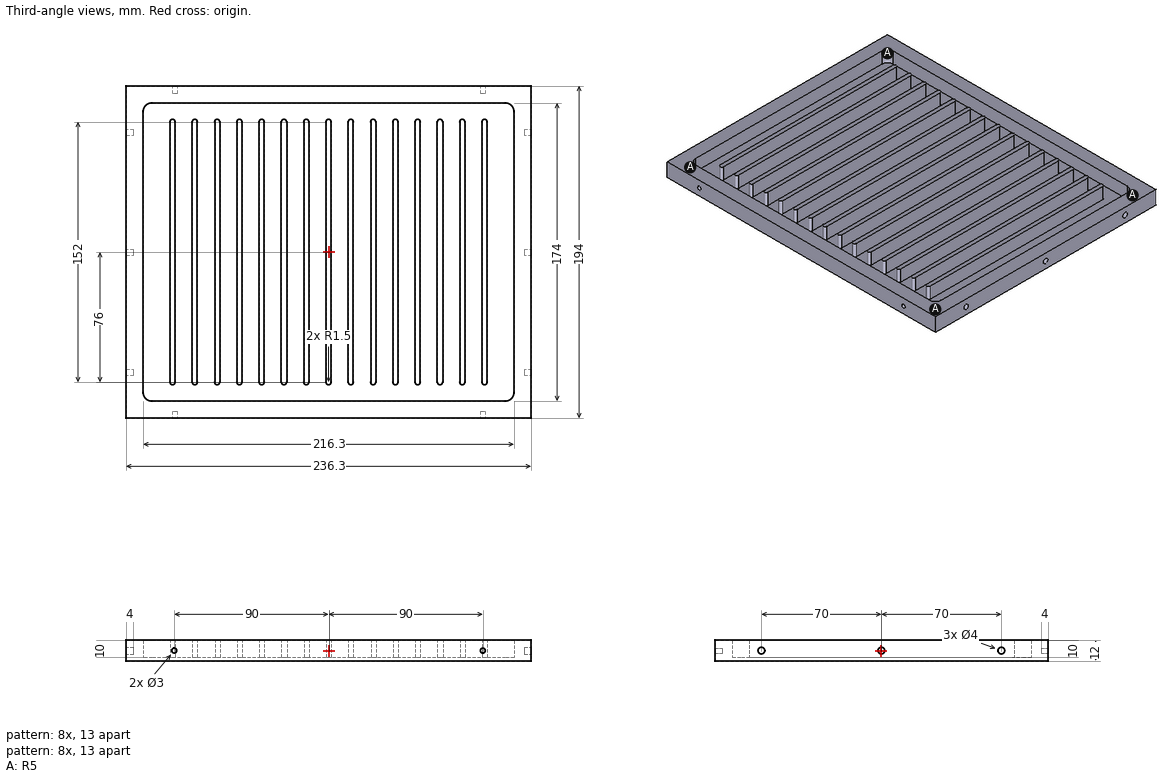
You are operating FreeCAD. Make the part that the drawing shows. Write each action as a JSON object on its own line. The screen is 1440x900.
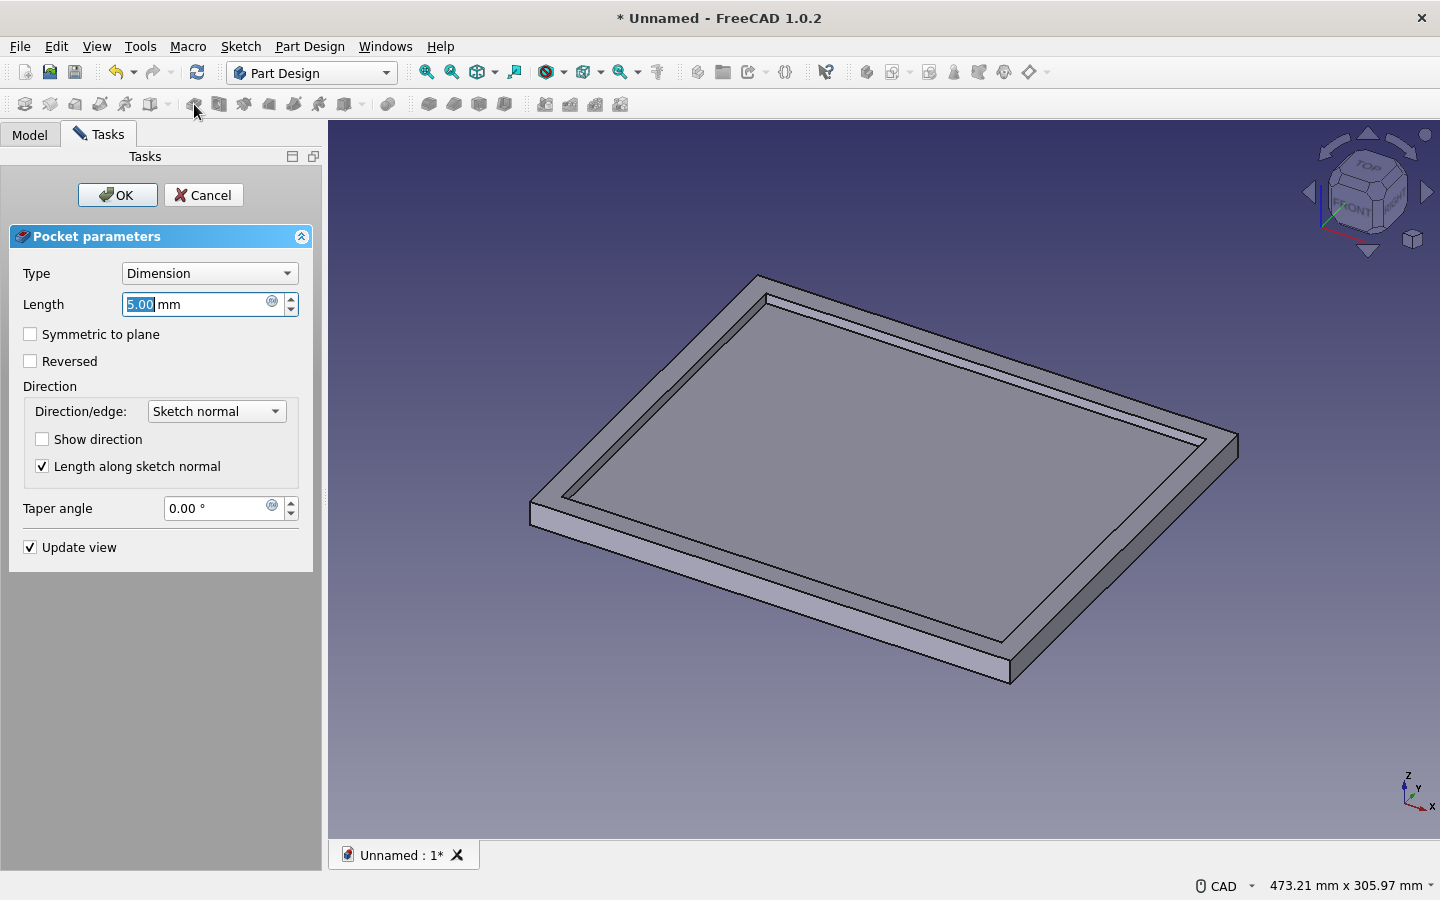
{"action": "type", "text": "10"}
{"action": "key", "text": "Tab"}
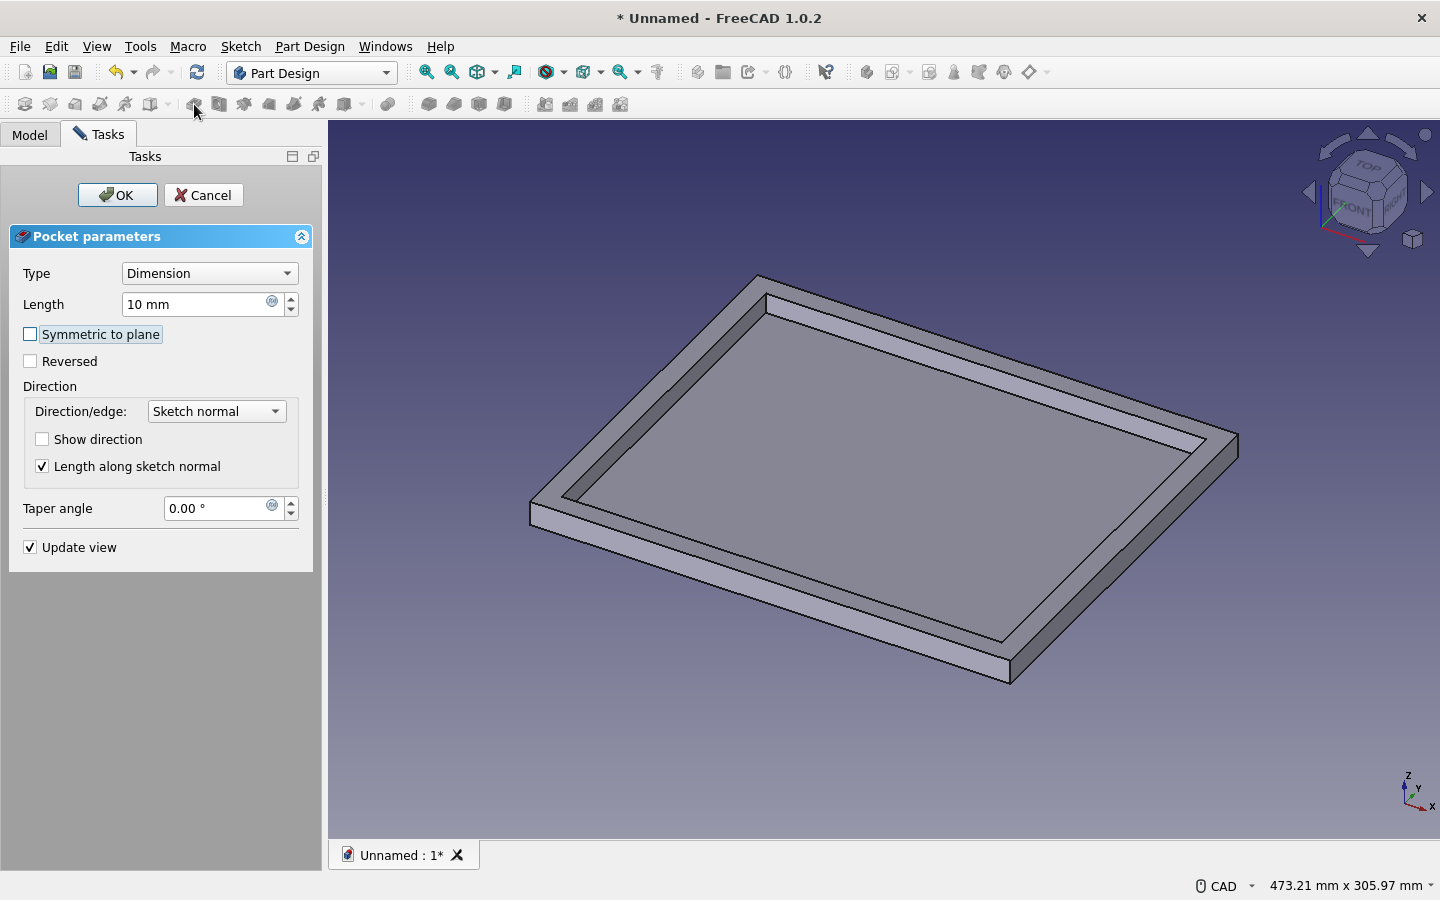
{"action": "left_click", "coordinate": [118, 195]}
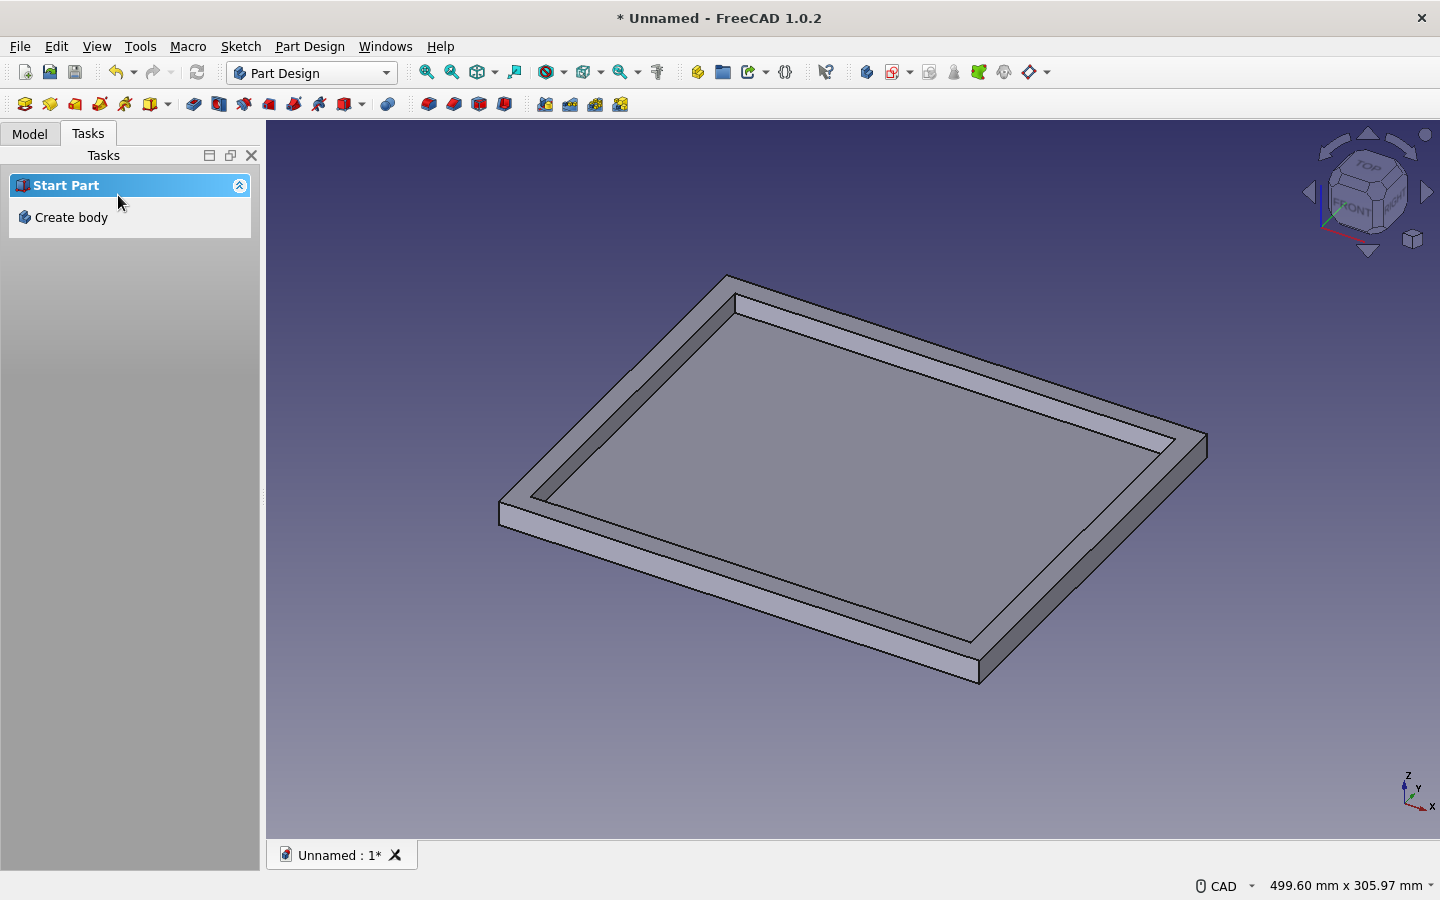
{"action": "left_click", "coordinate": [853, 486]}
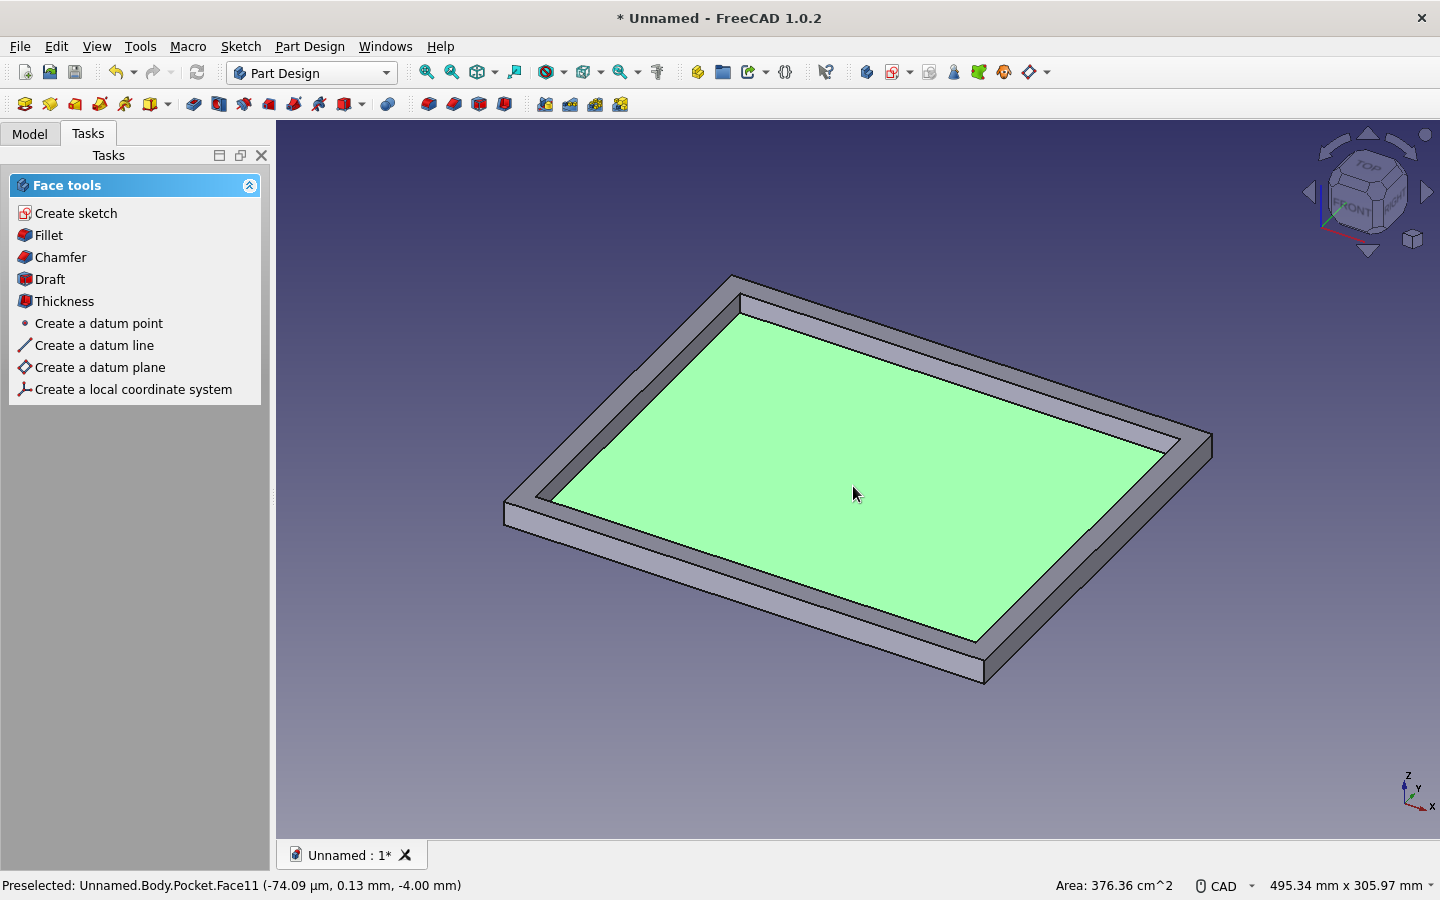
{"action": "left_click", "coordinate": [892, 72]}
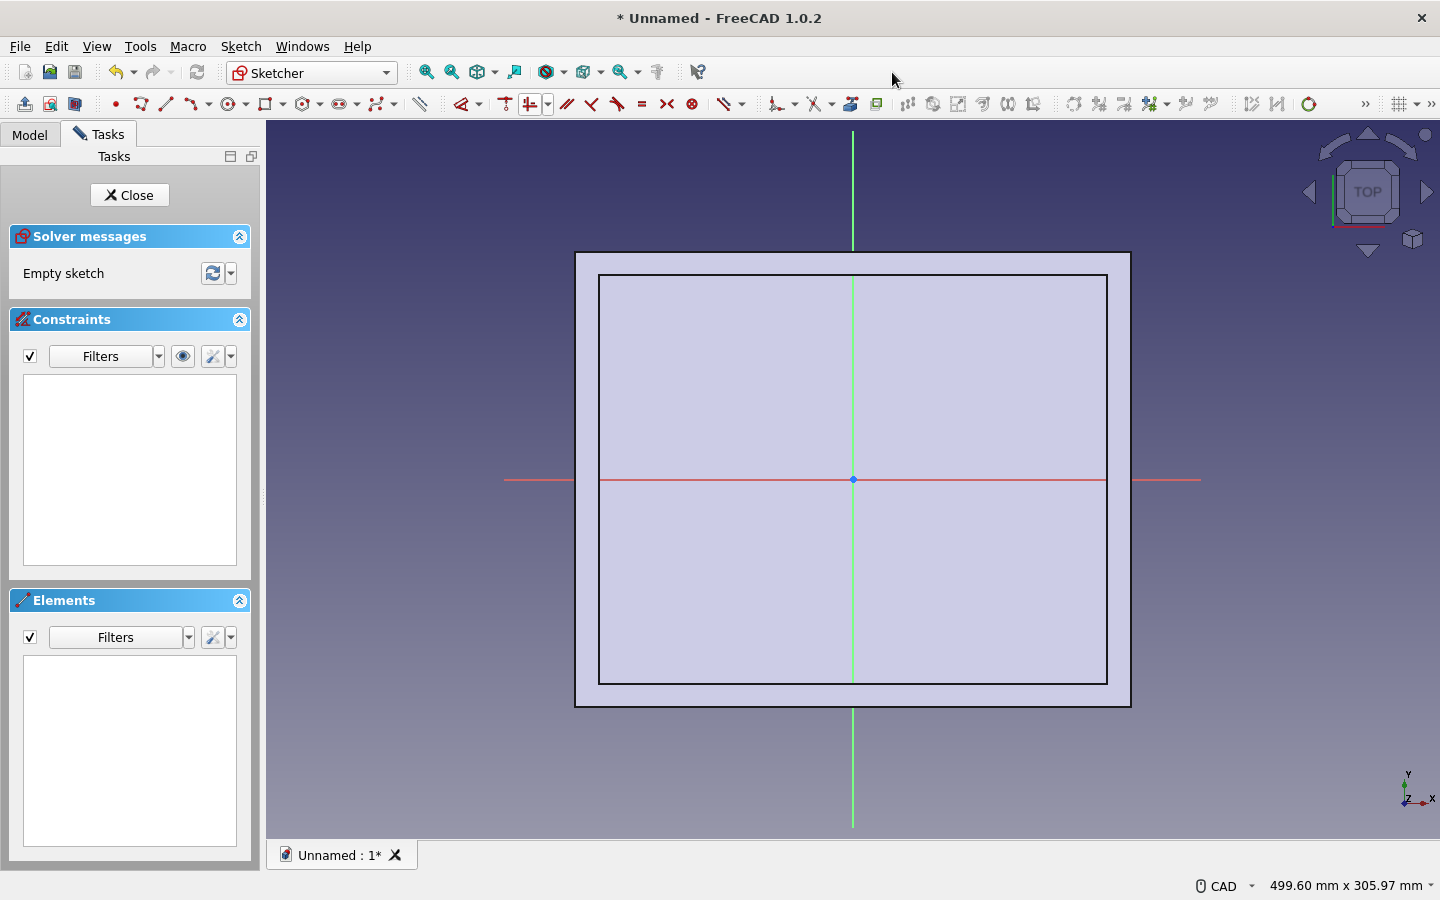
{"action": "left_click", "coordinate": [338, 104]}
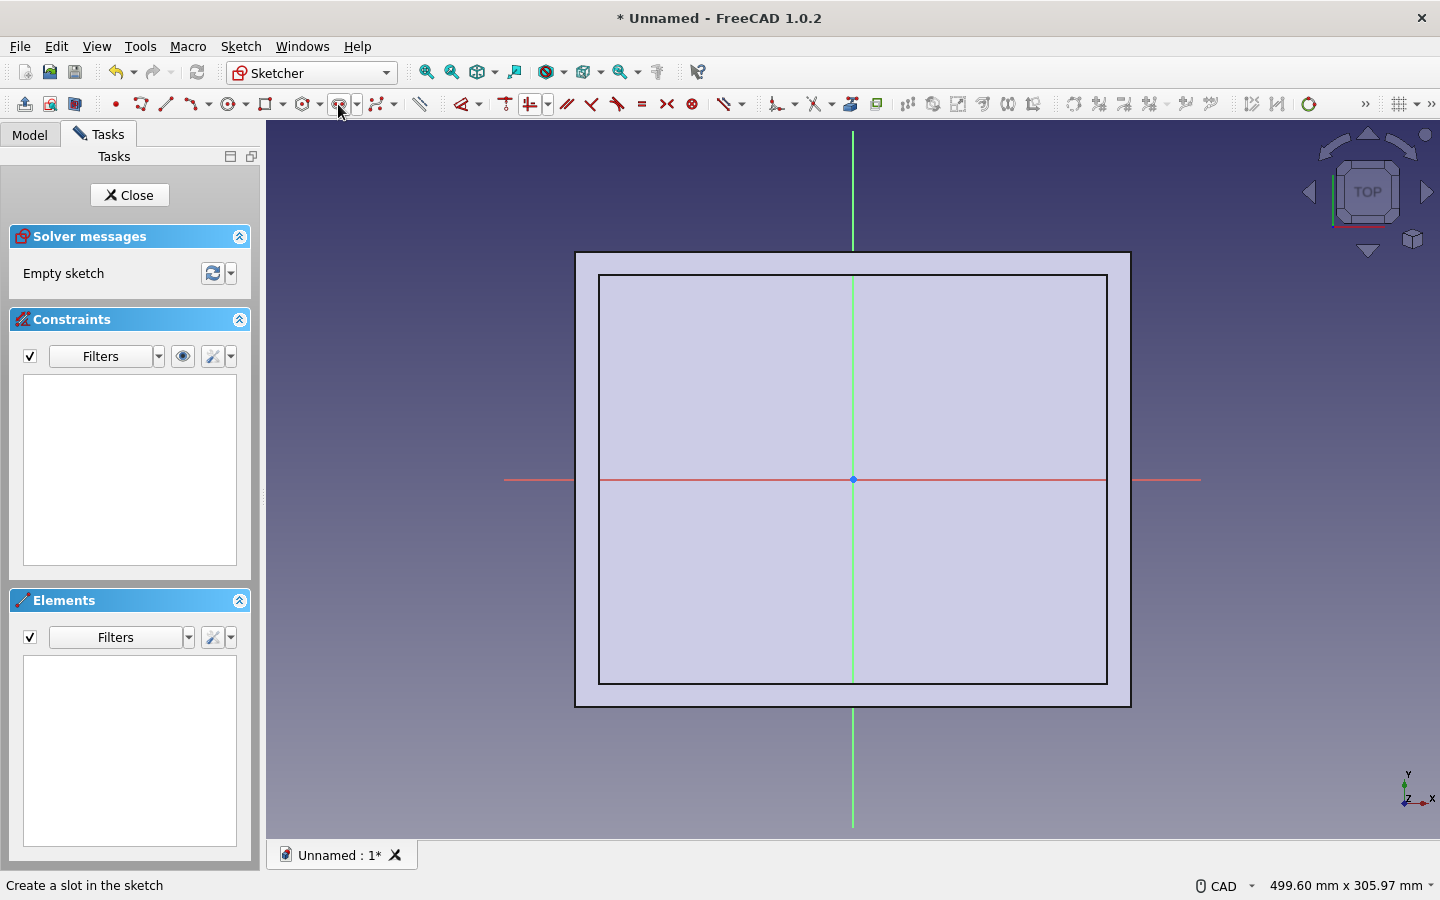
{"action": "scroll", "coordinate": [853, 658], "scroll_direction": "up", "scroll_amount": 10}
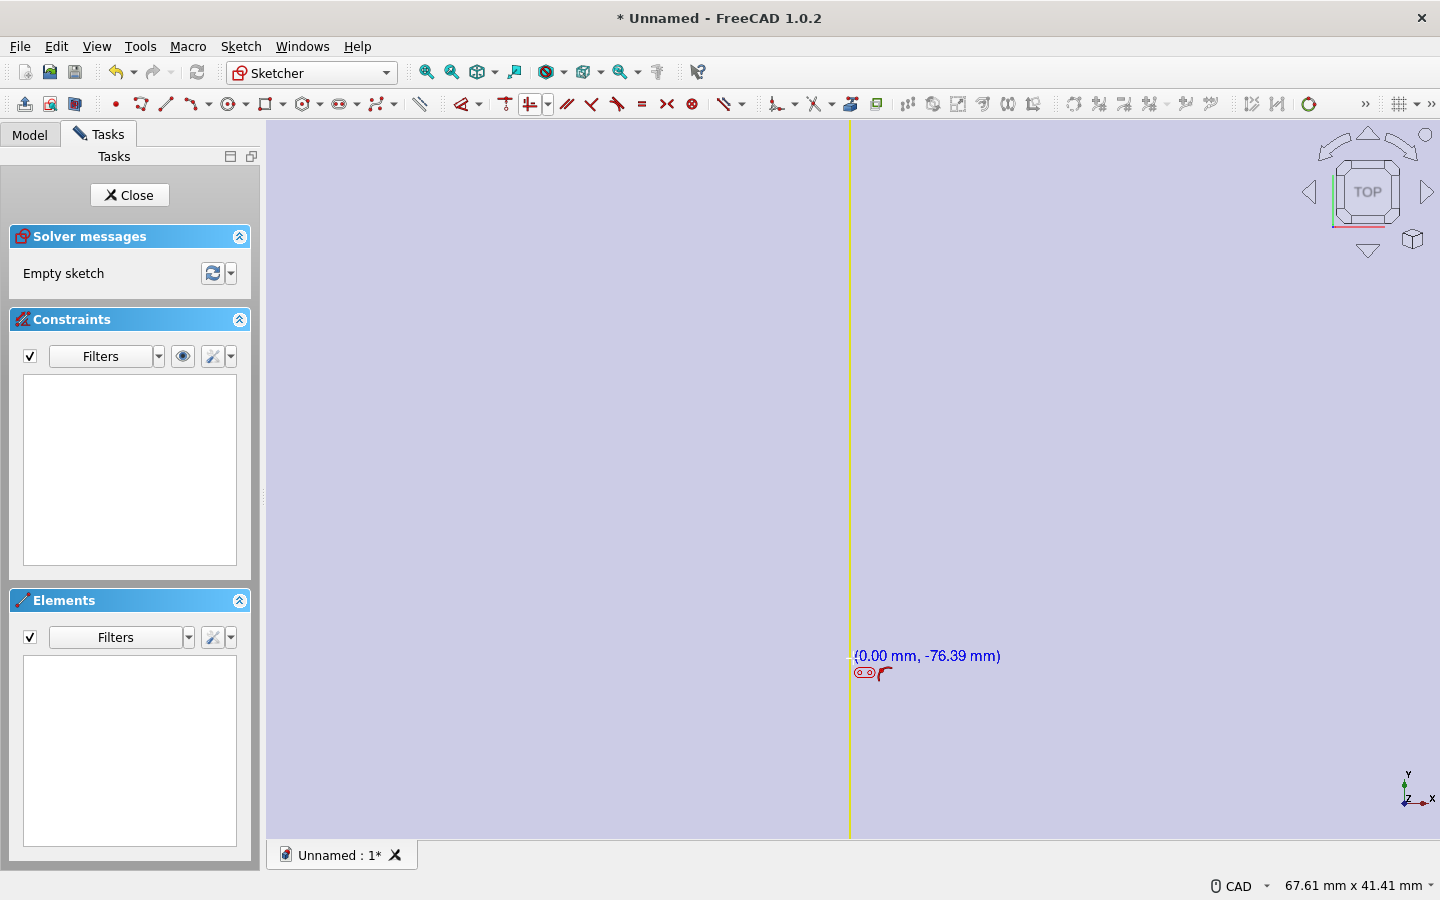
{"action": "scroll", "coordinate": [772, 706], "scroll_direction": "down", "scroll_amount": 9}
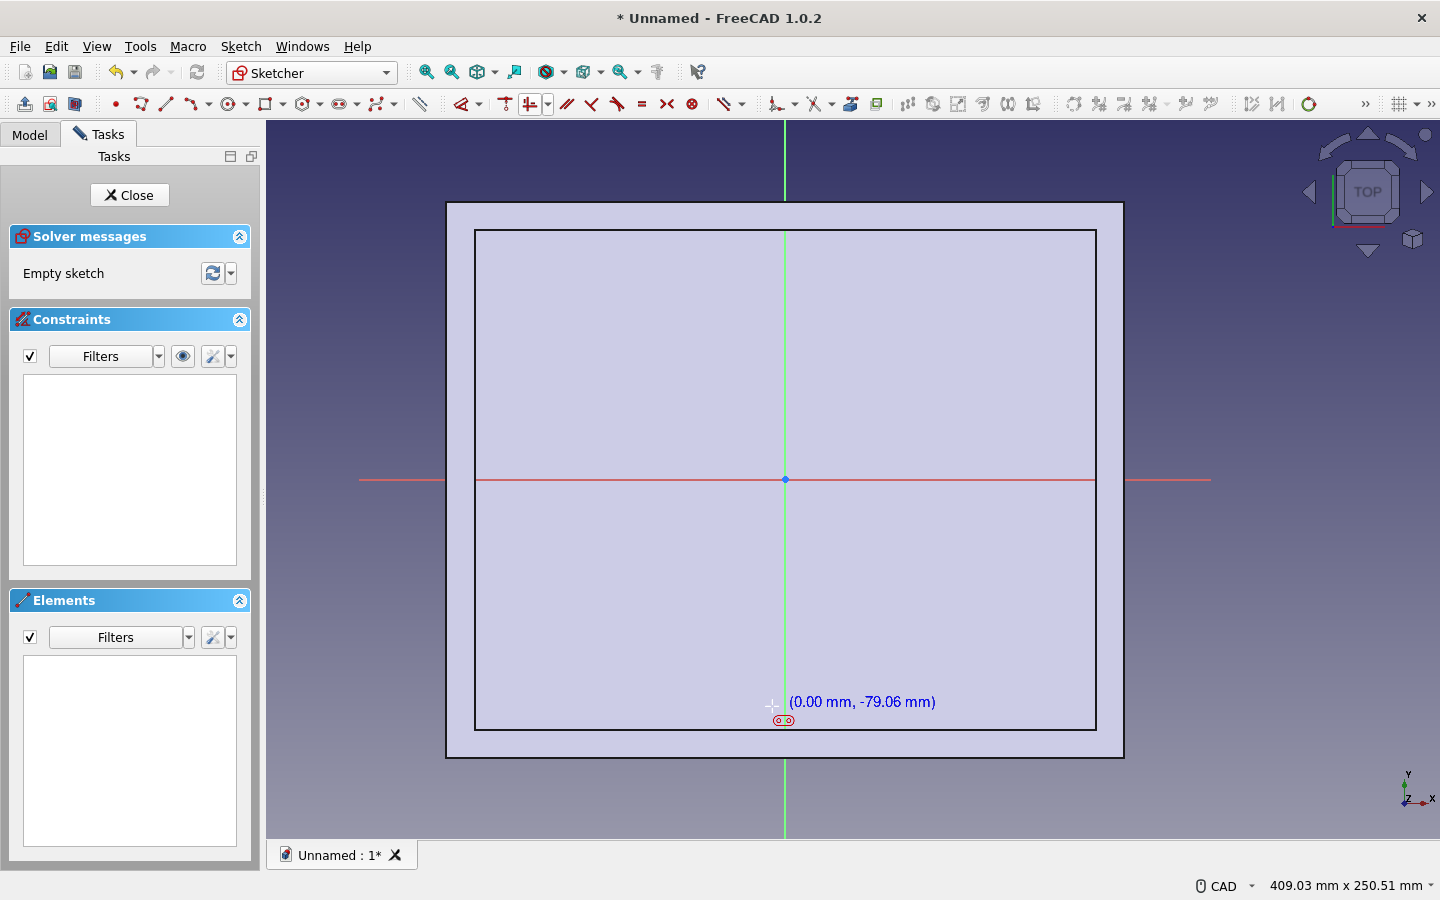
{"action": "left_click", "coordinate": [785, 698]}